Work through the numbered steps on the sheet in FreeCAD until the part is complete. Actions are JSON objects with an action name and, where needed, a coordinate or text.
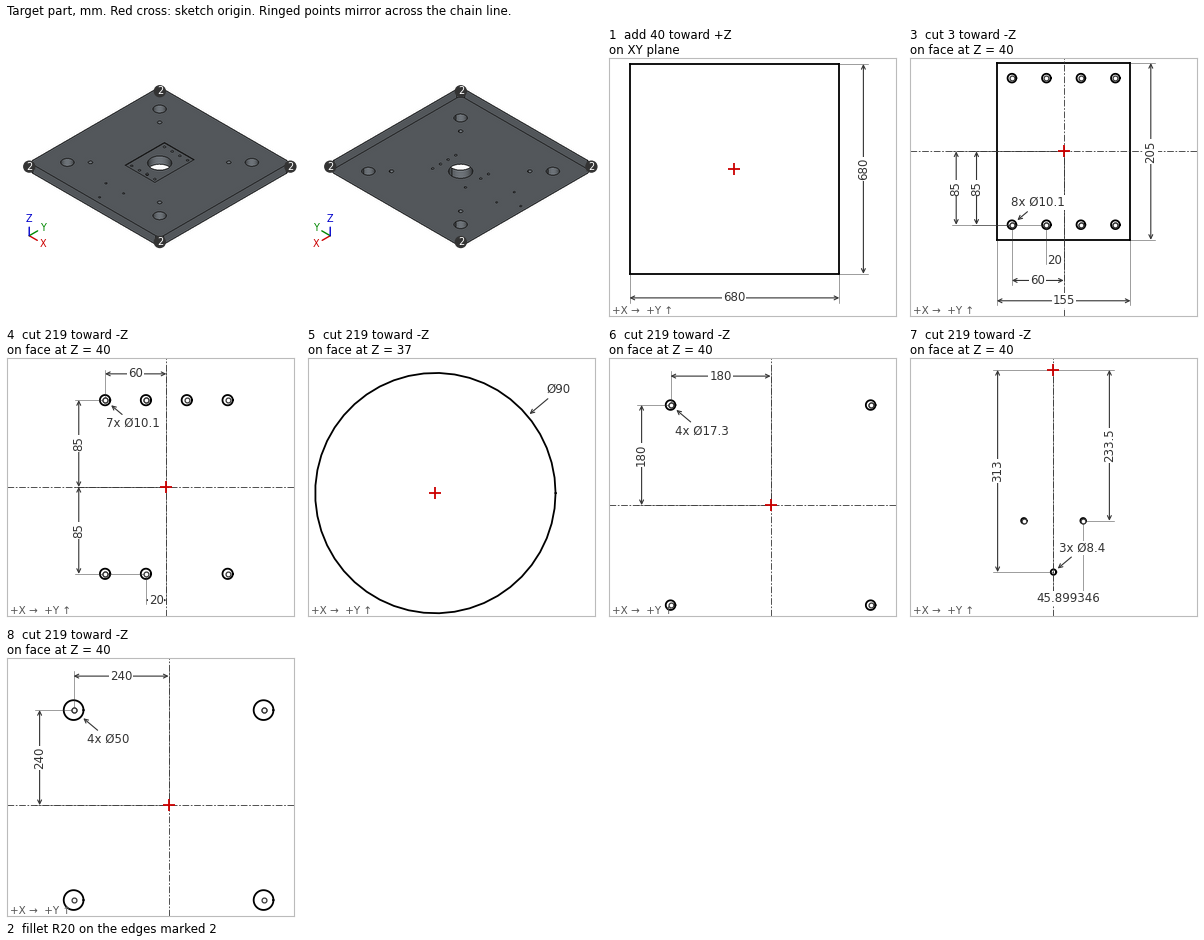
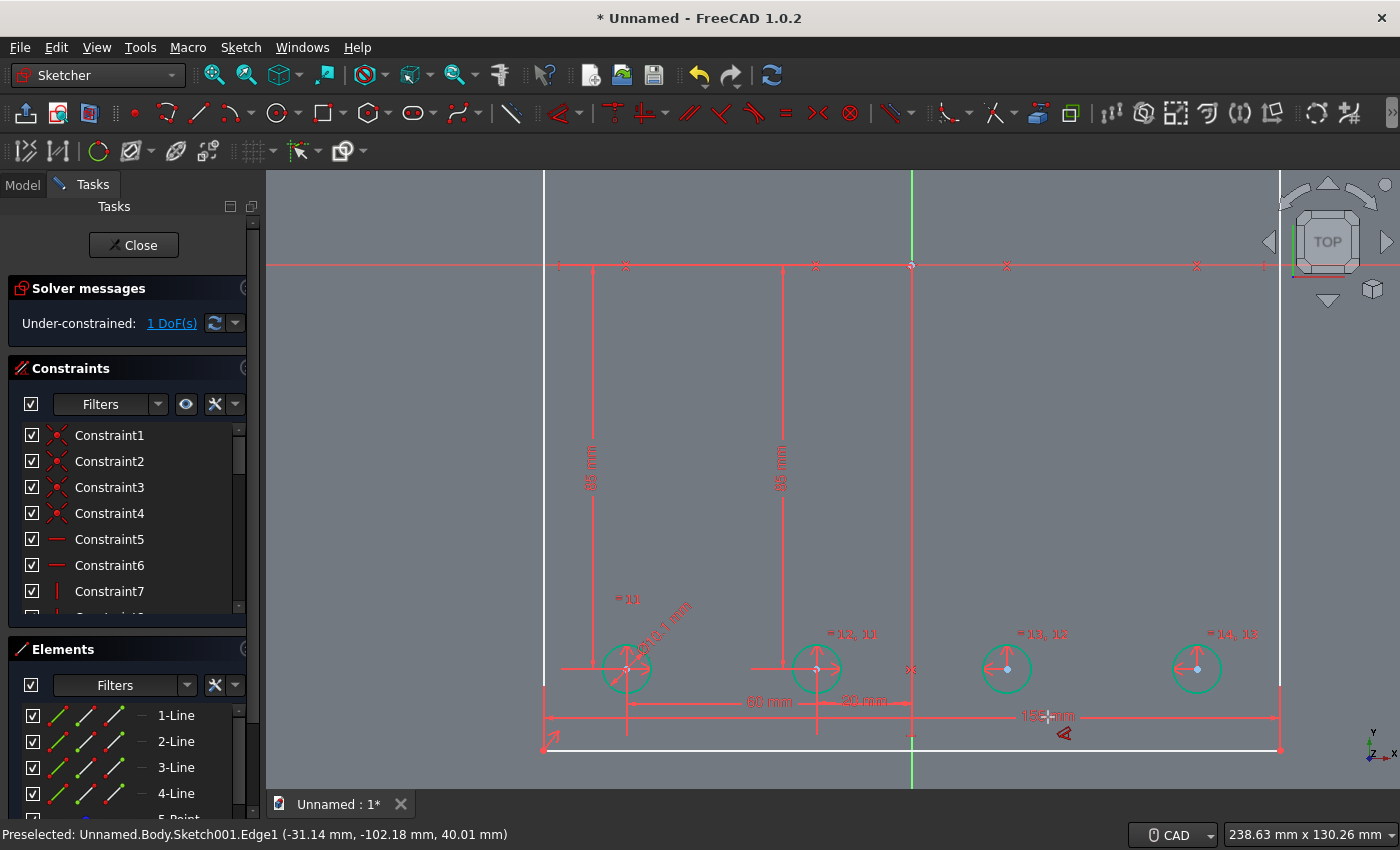
{"action": "scroll", "coordinate": [644, 654], "scroll_direction": "down", "scroll_amount": 4}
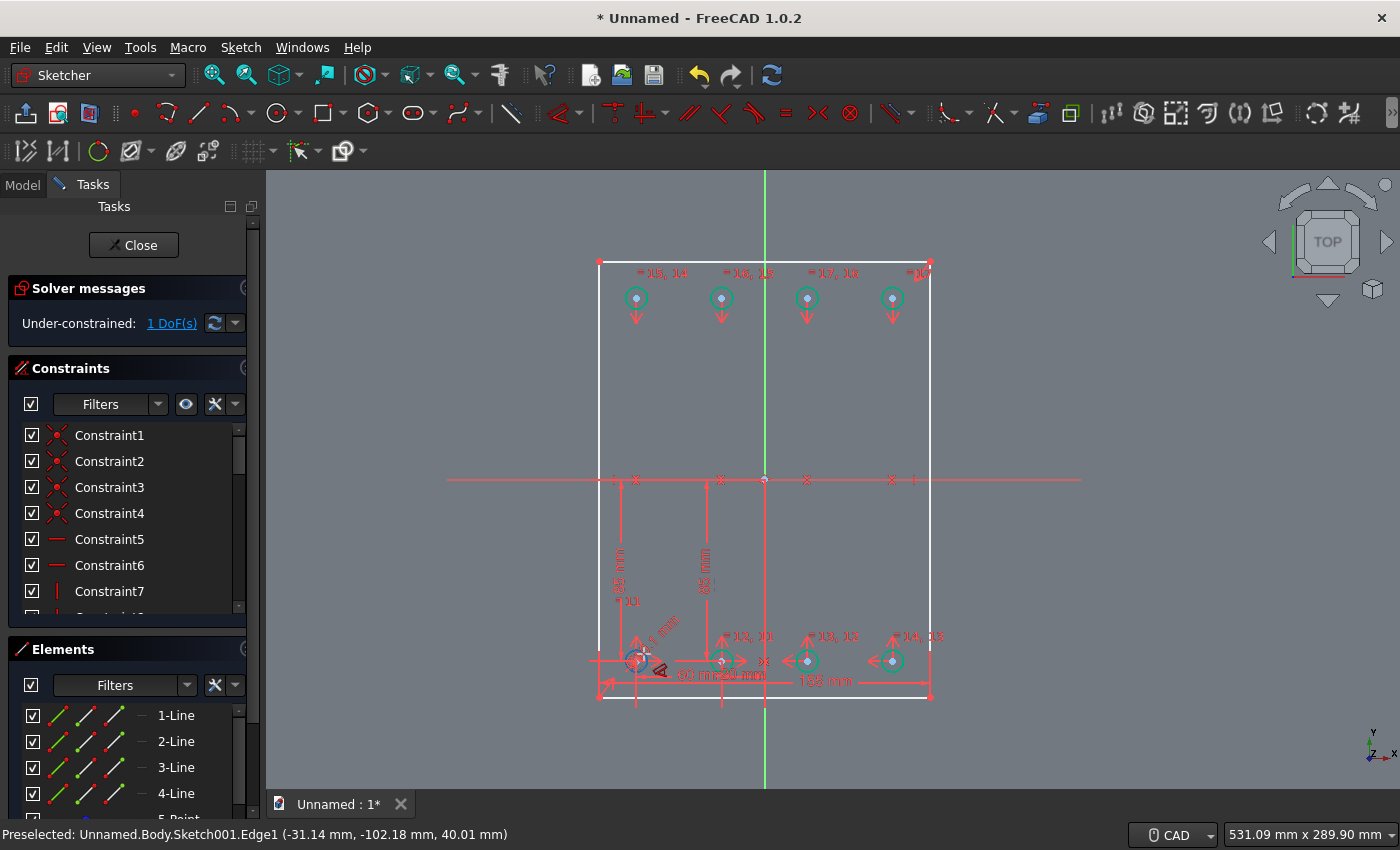
{"action": "left_click", "coordinate": [930, 567]}
{"action": "left_click", "coordinate": [964, 379]}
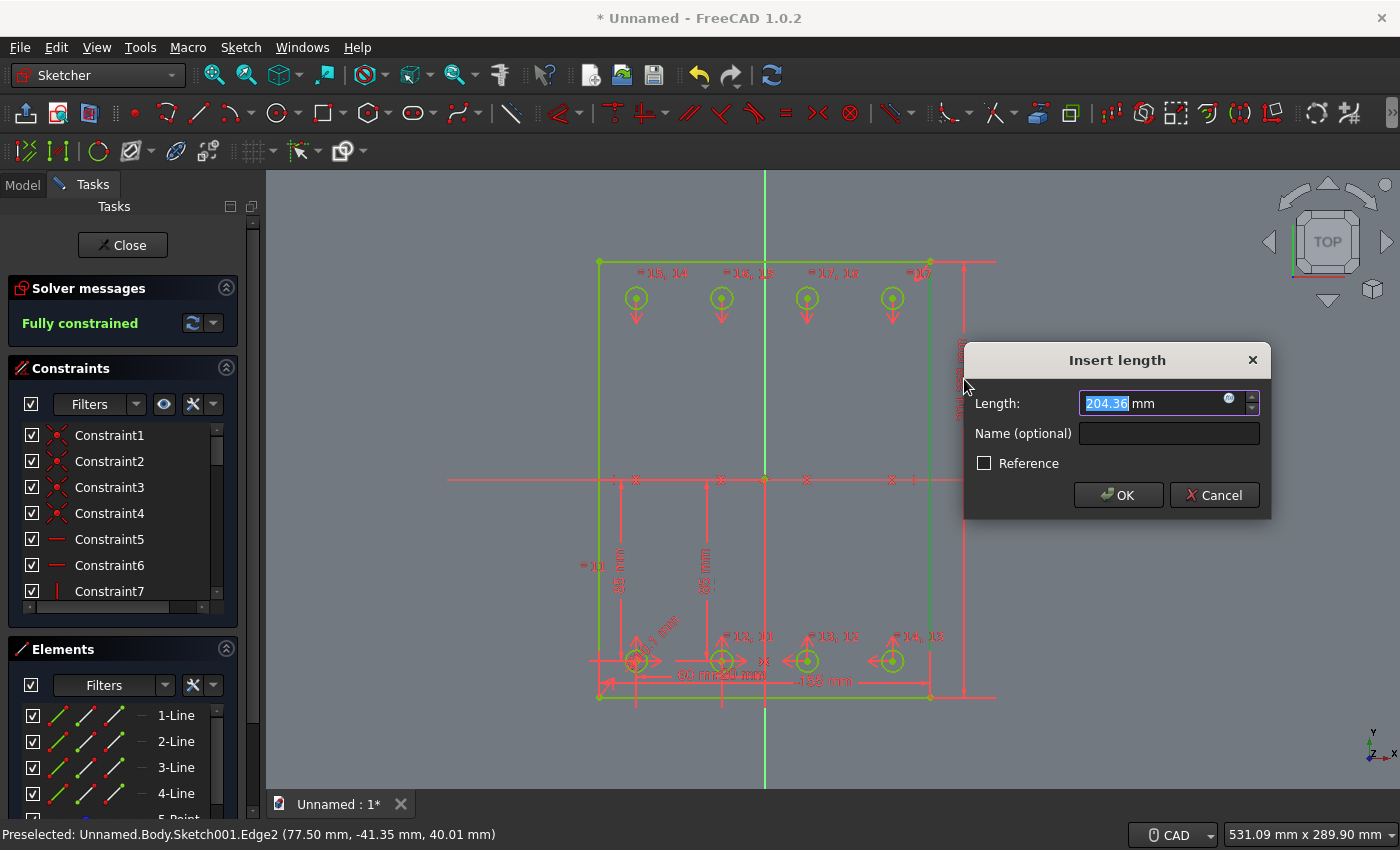
{"action": "type", "text": "205"}
{"action": "key", "text": "Return"}
{"action": "key", "text": "Escape"}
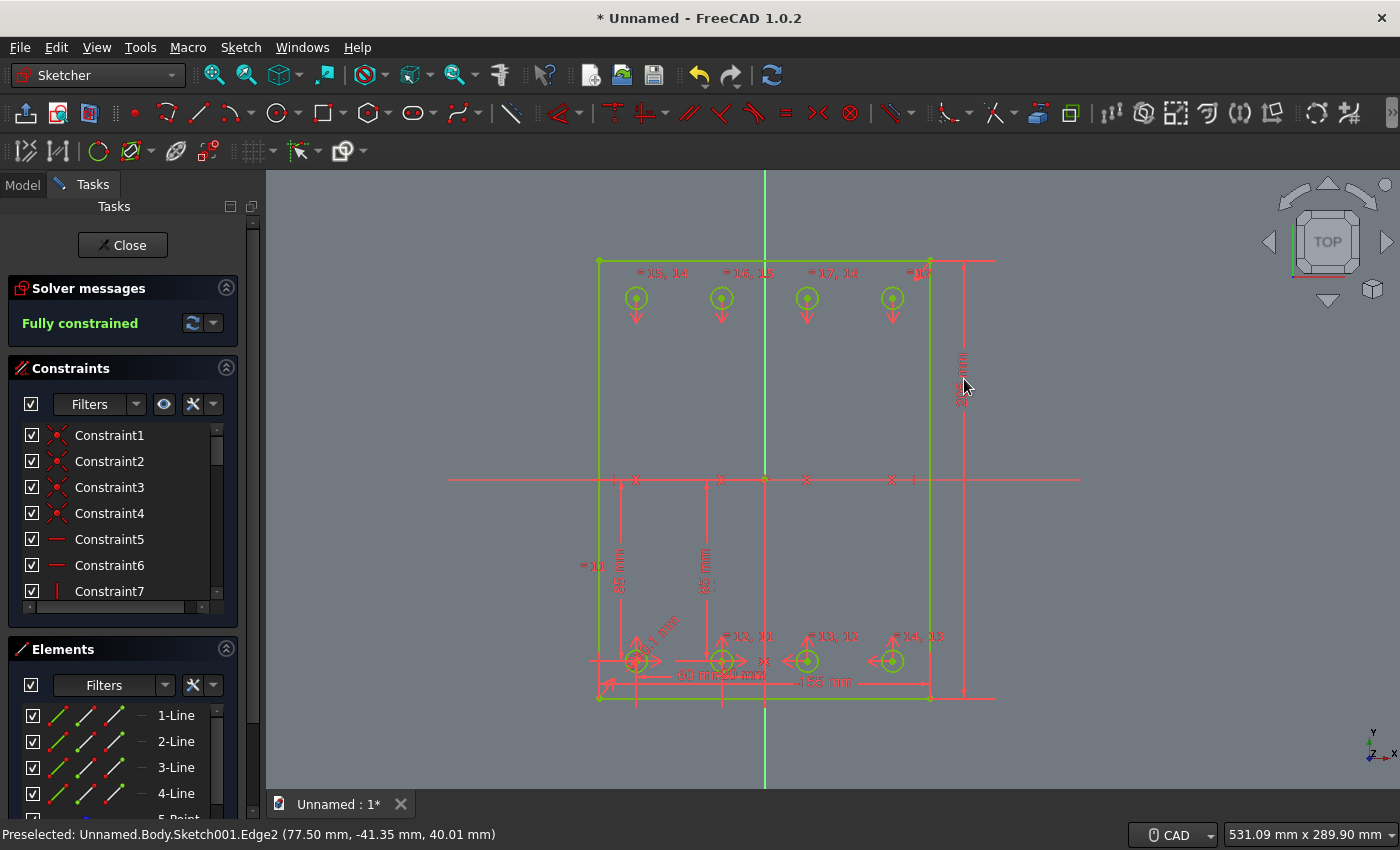
{"action": "left_click", "coordinate": [123, 245]}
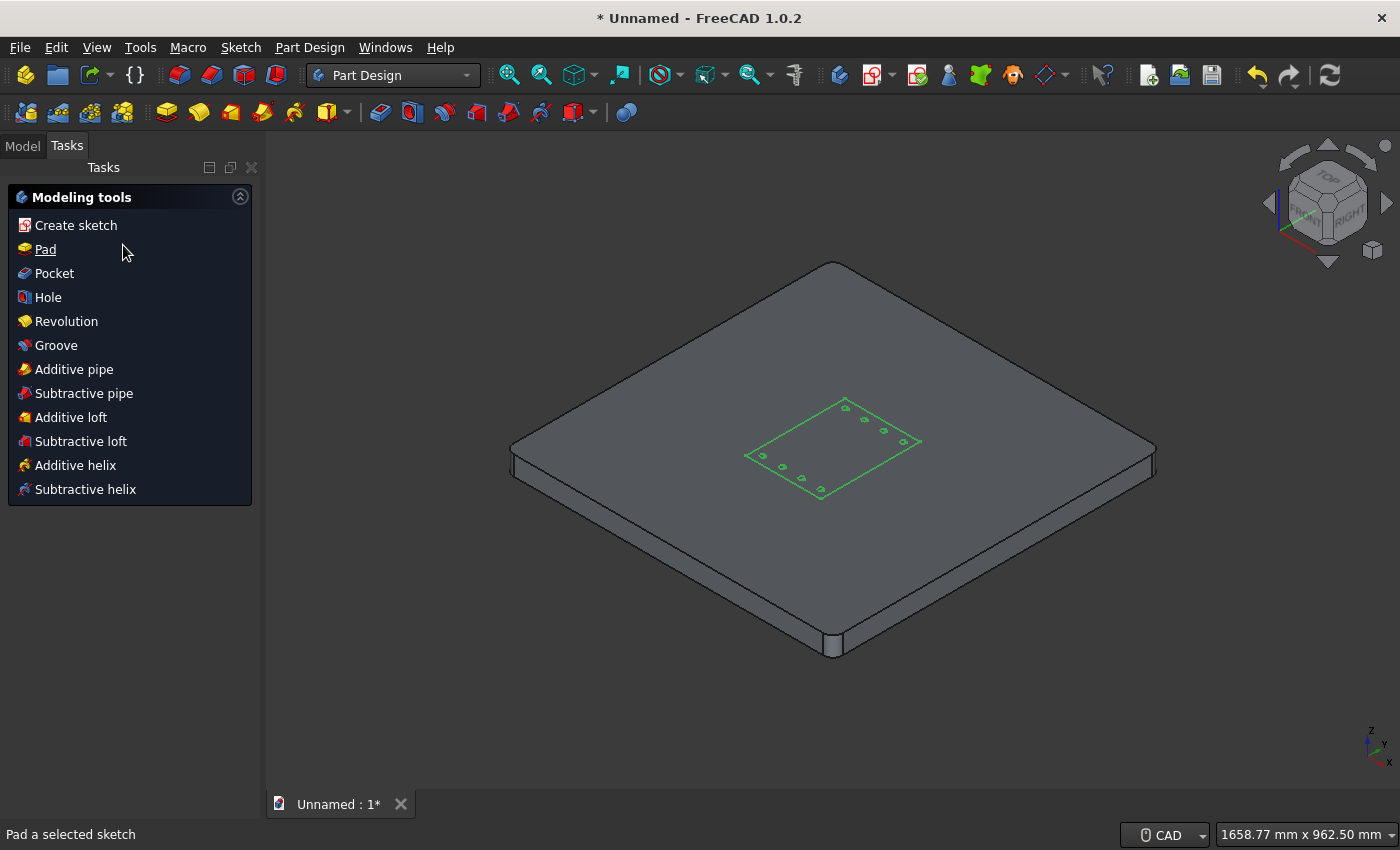
{"action": "left_click", "coordinate": [382, 112]}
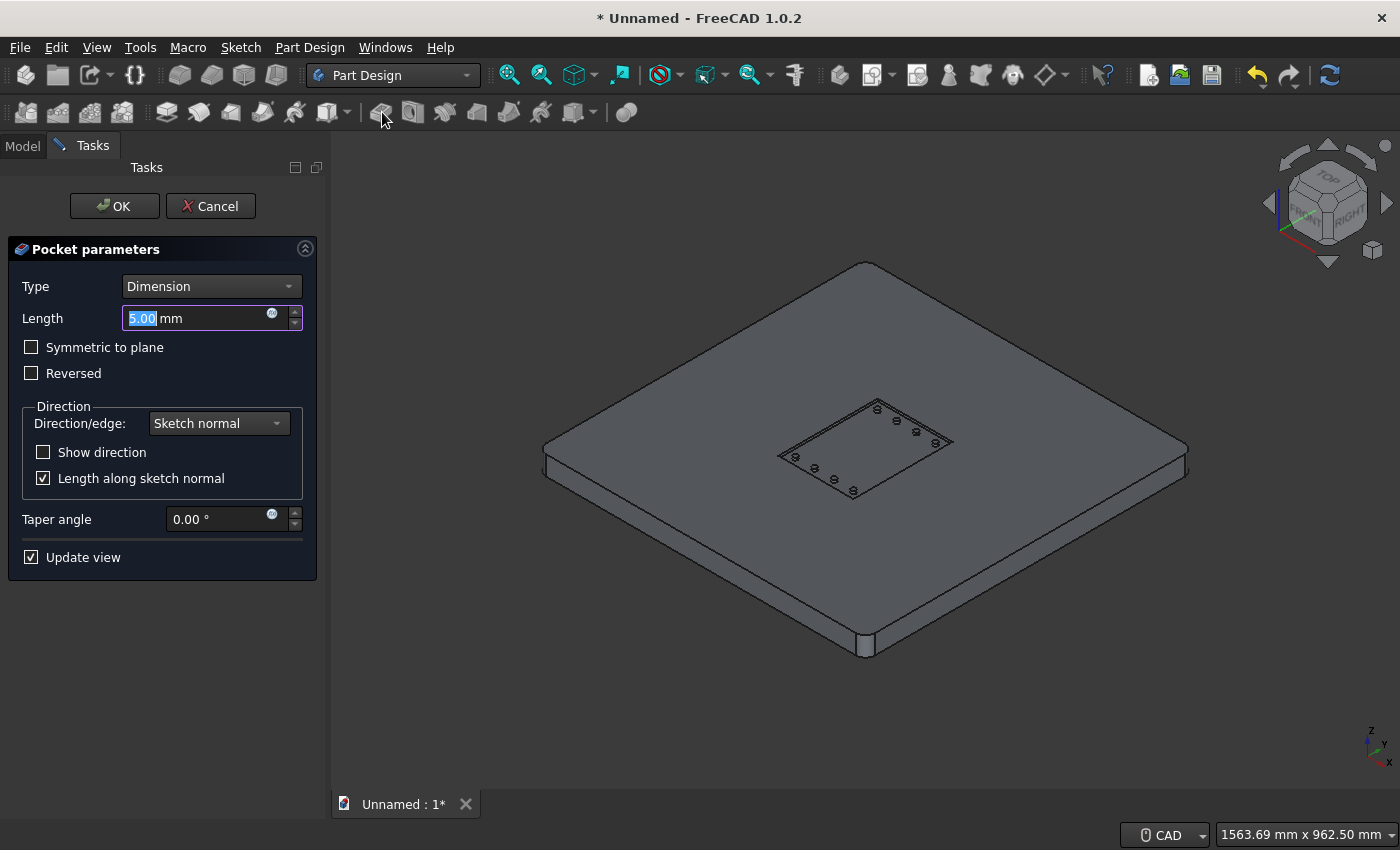
{"action": "type", "text": "3"}
{"action": "key", "text": "Tab"}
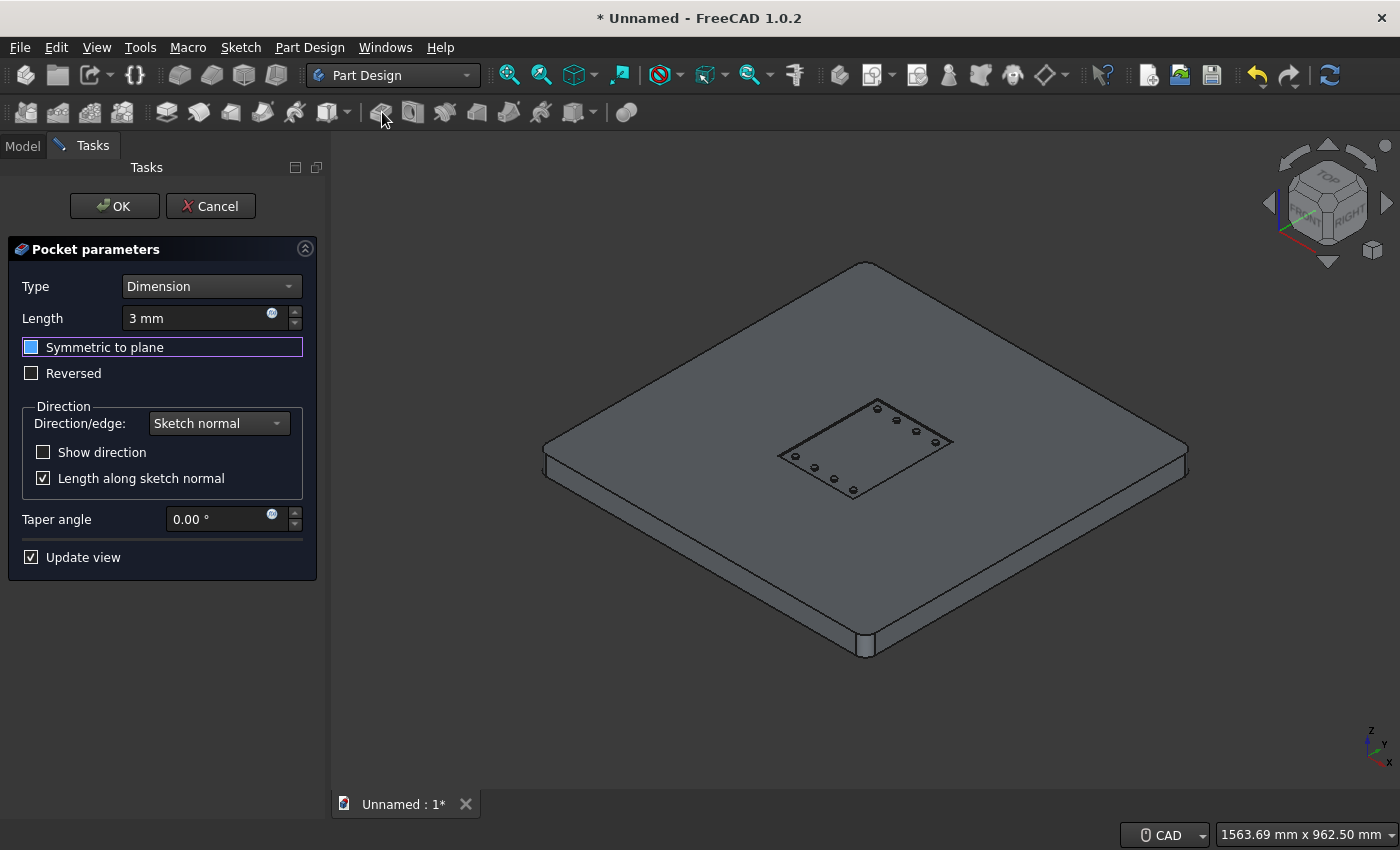
{"action": "left_click", "coordinate": [115, 206]}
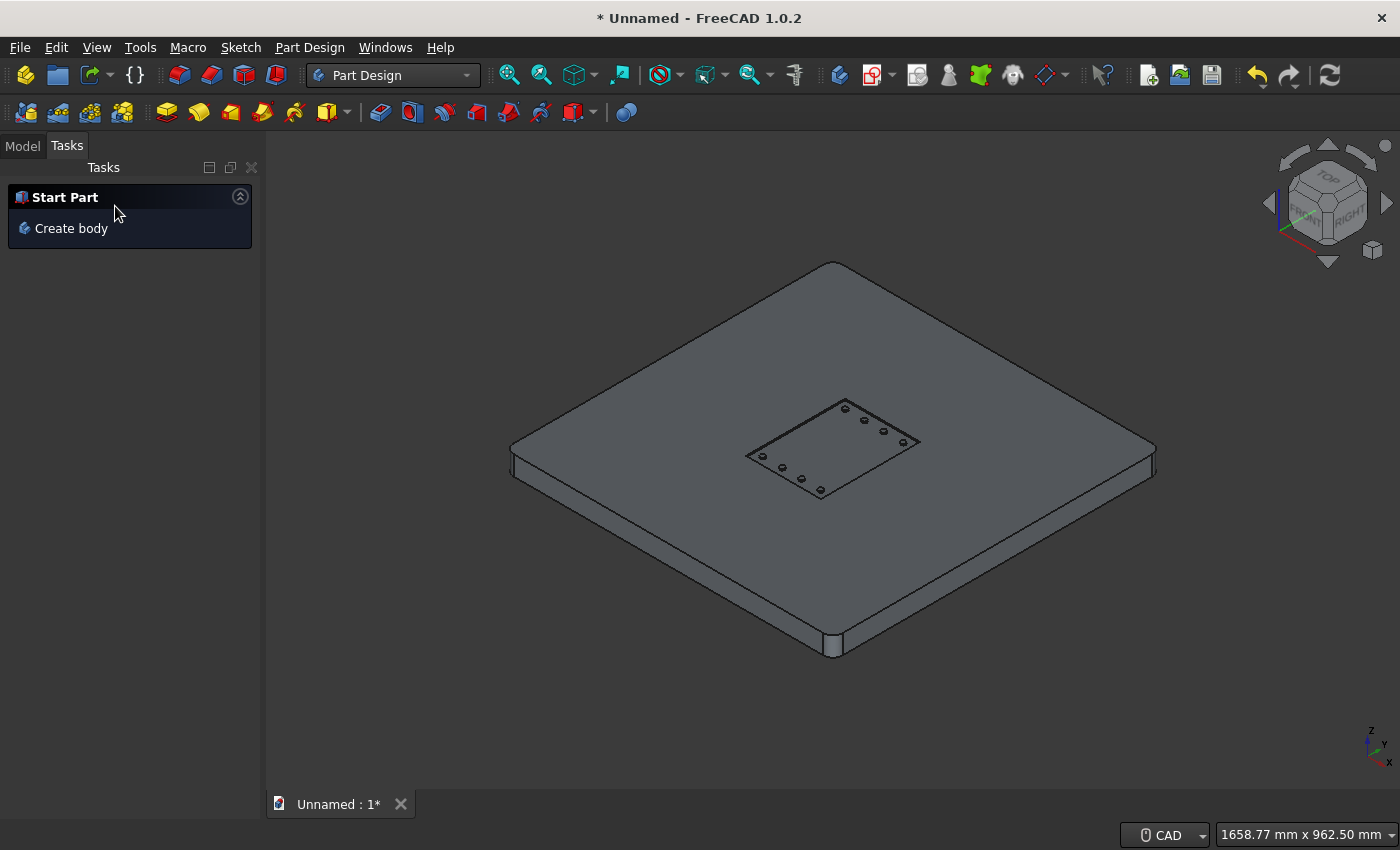
{"action": "left_click", "coordinate": [645, 448]}